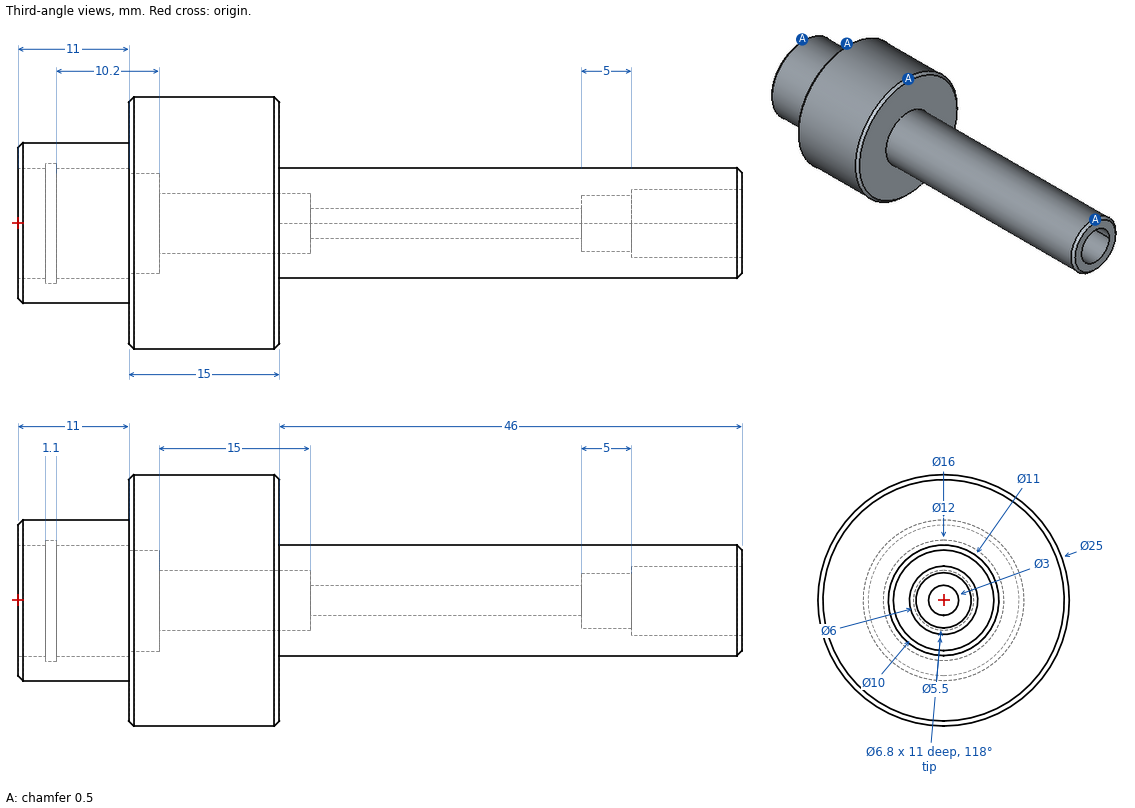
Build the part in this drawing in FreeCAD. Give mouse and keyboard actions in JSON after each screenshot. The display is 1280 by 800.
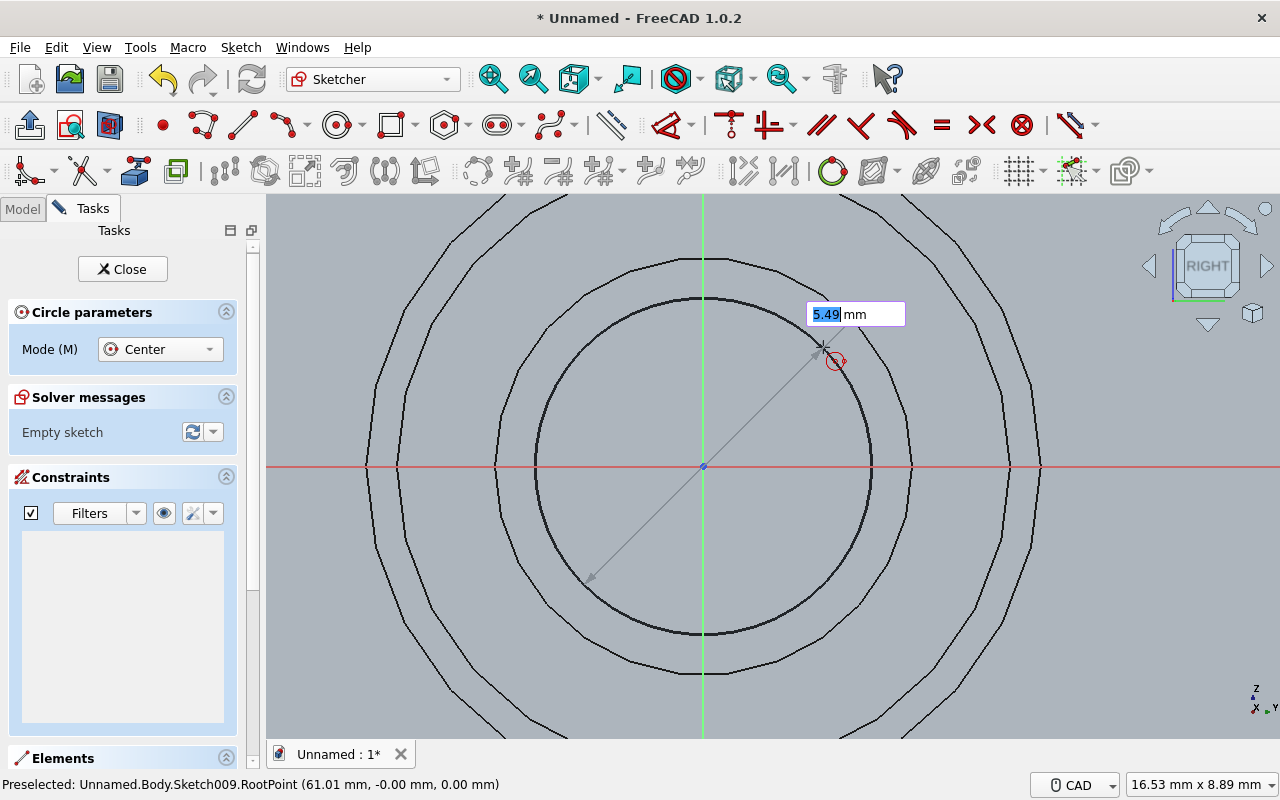
{"action": "type", "text": "5.5"}
{"action": "key", "text": "Return"}
{"action": "key", "text": "Escape"}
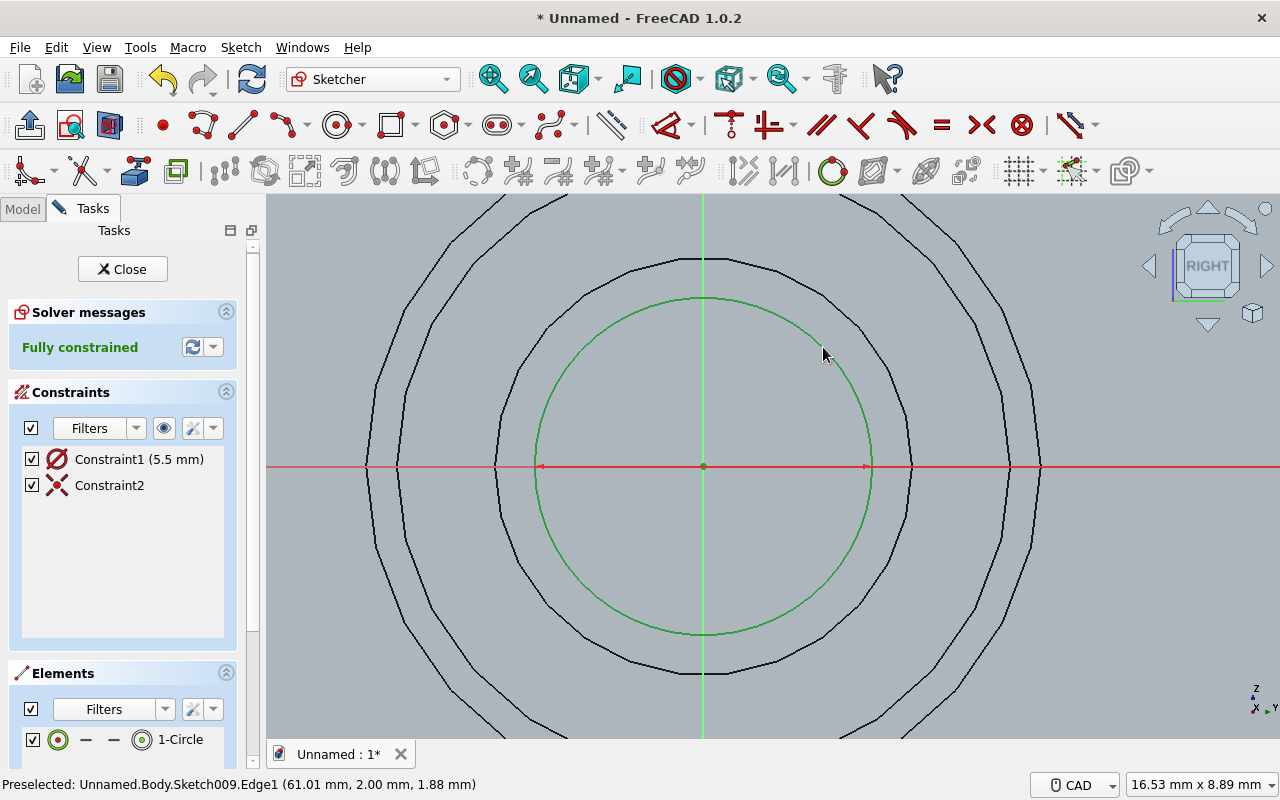
{"action": "left_click", "coordinate": [123, 269]}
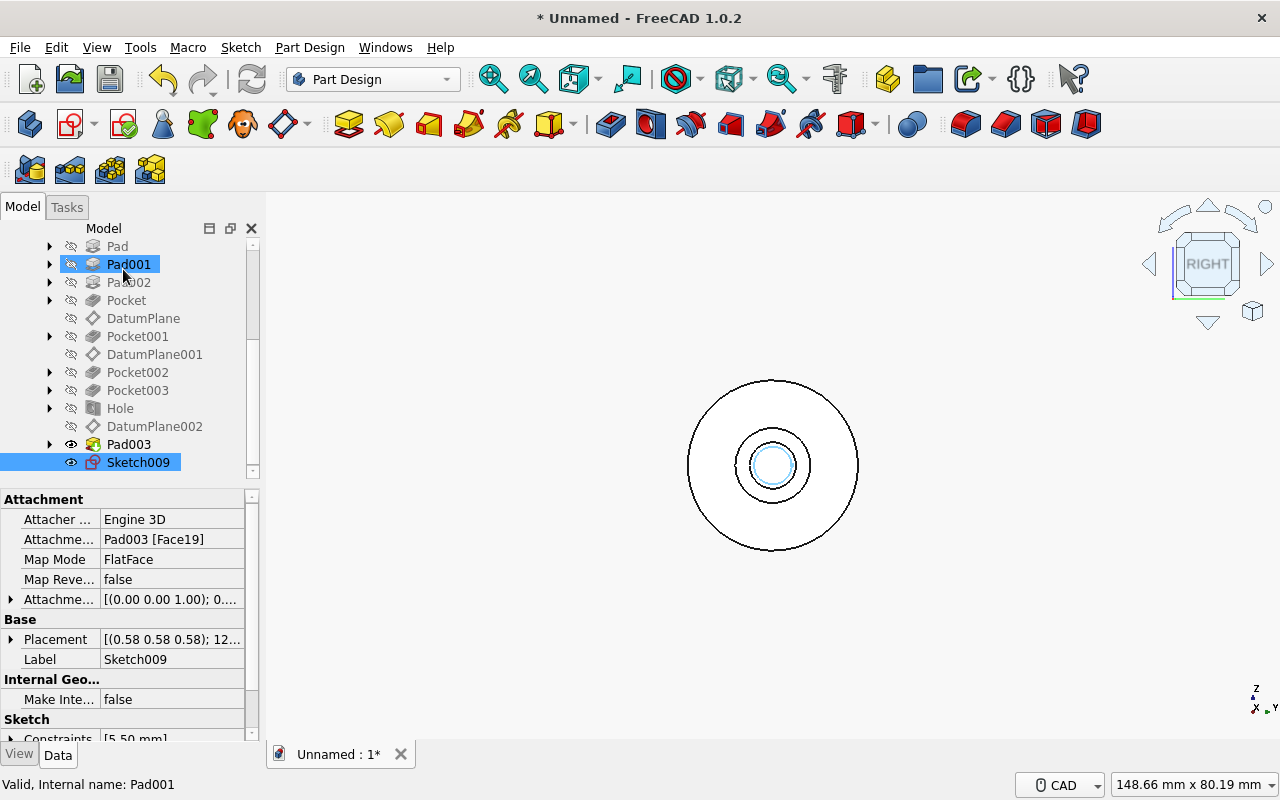
{"action": "left_click", "coordinate": [612, 124]}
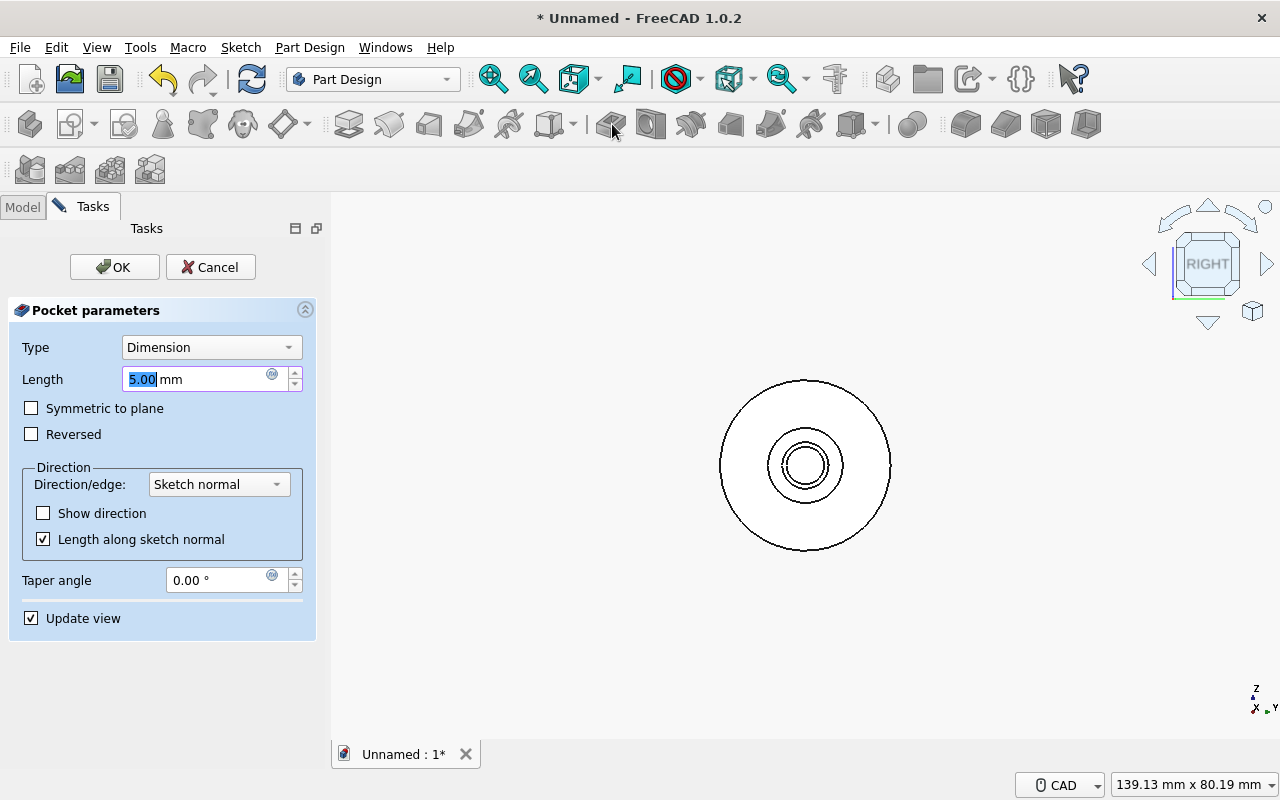
{"action": "type", "text": "5"}
{"action": "key", "text": "Tab"}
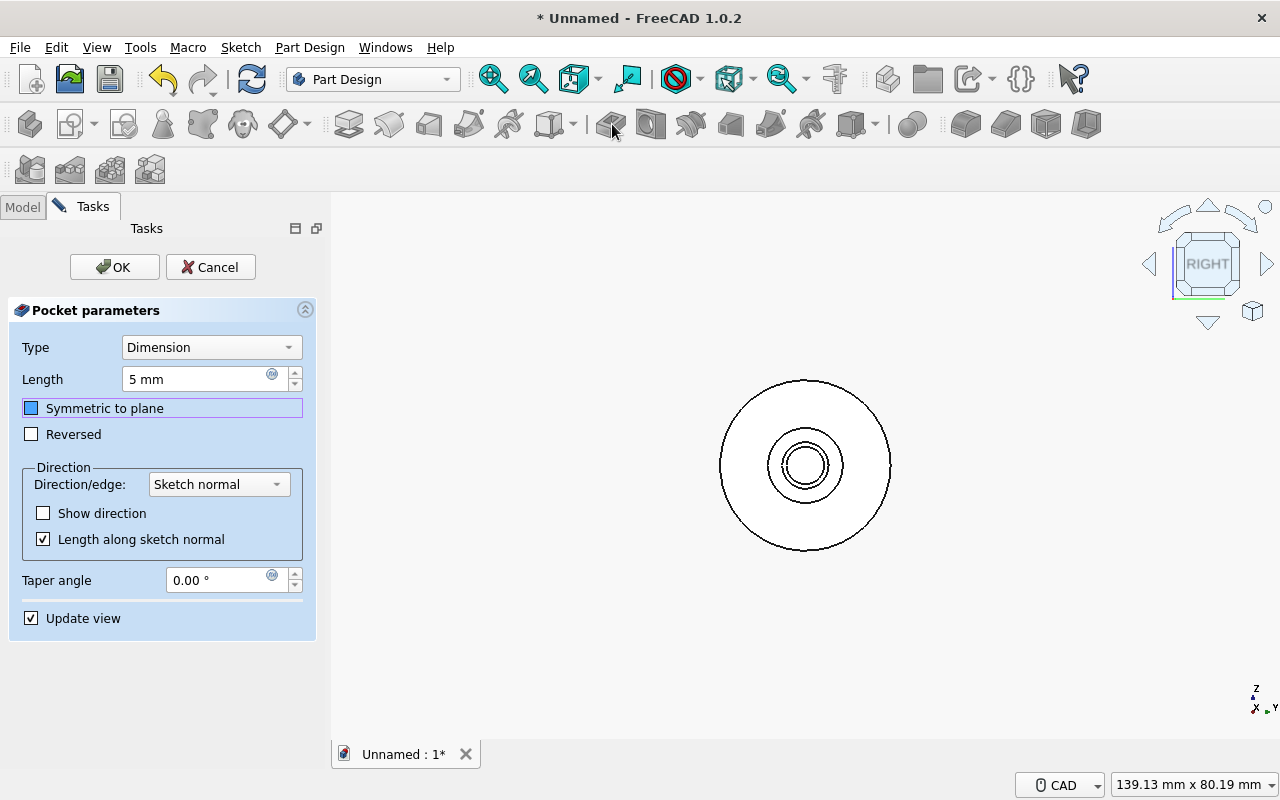
{"action": "left_click", "coordinate": [115, 267]}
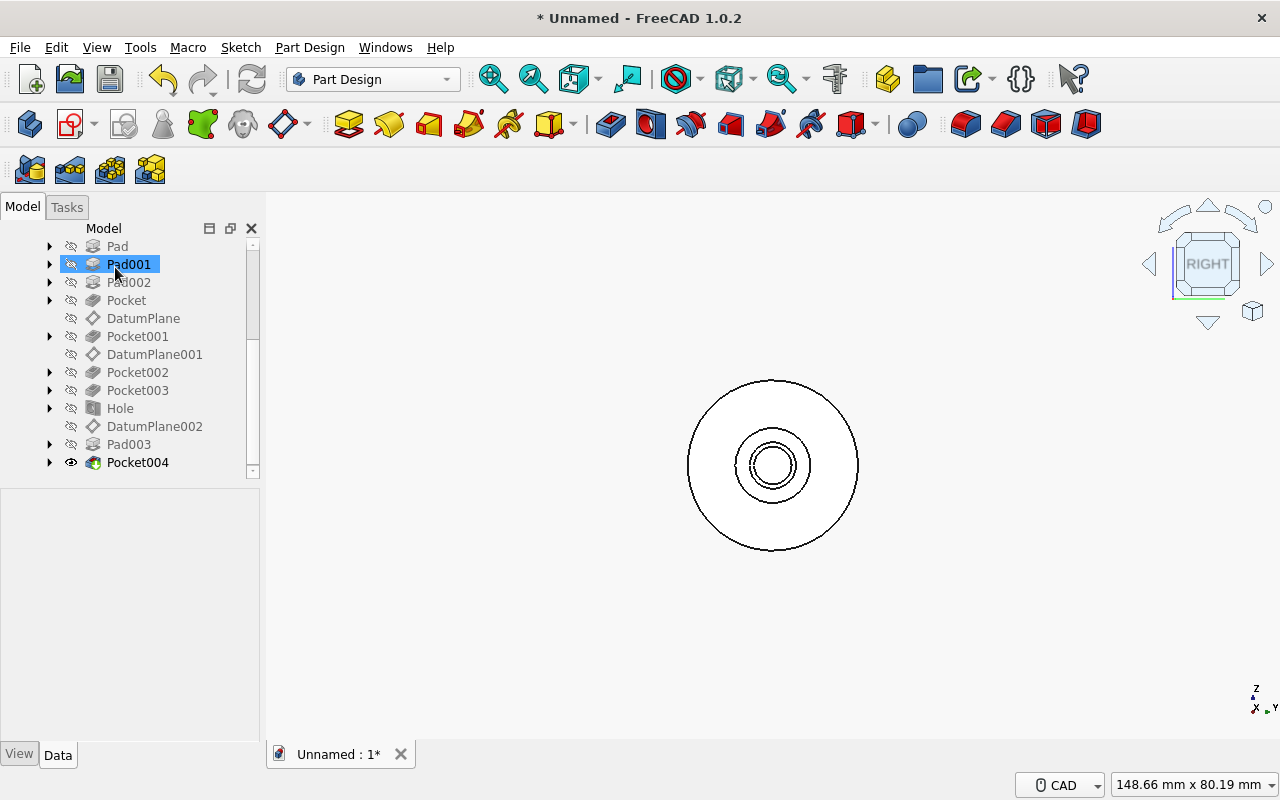
{"action": "left_click", "coordinate": [494, 80]}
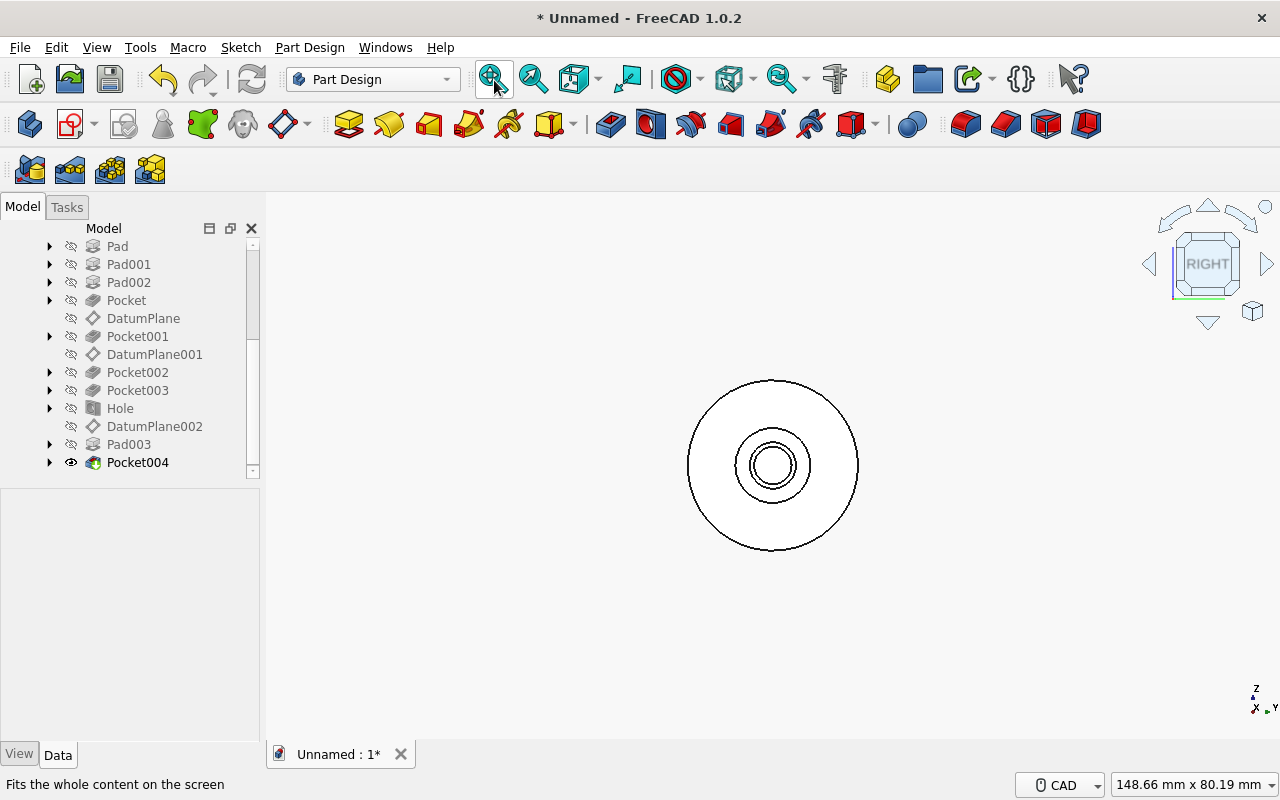
{"action": "left_click", "coordinate": [773, 464]}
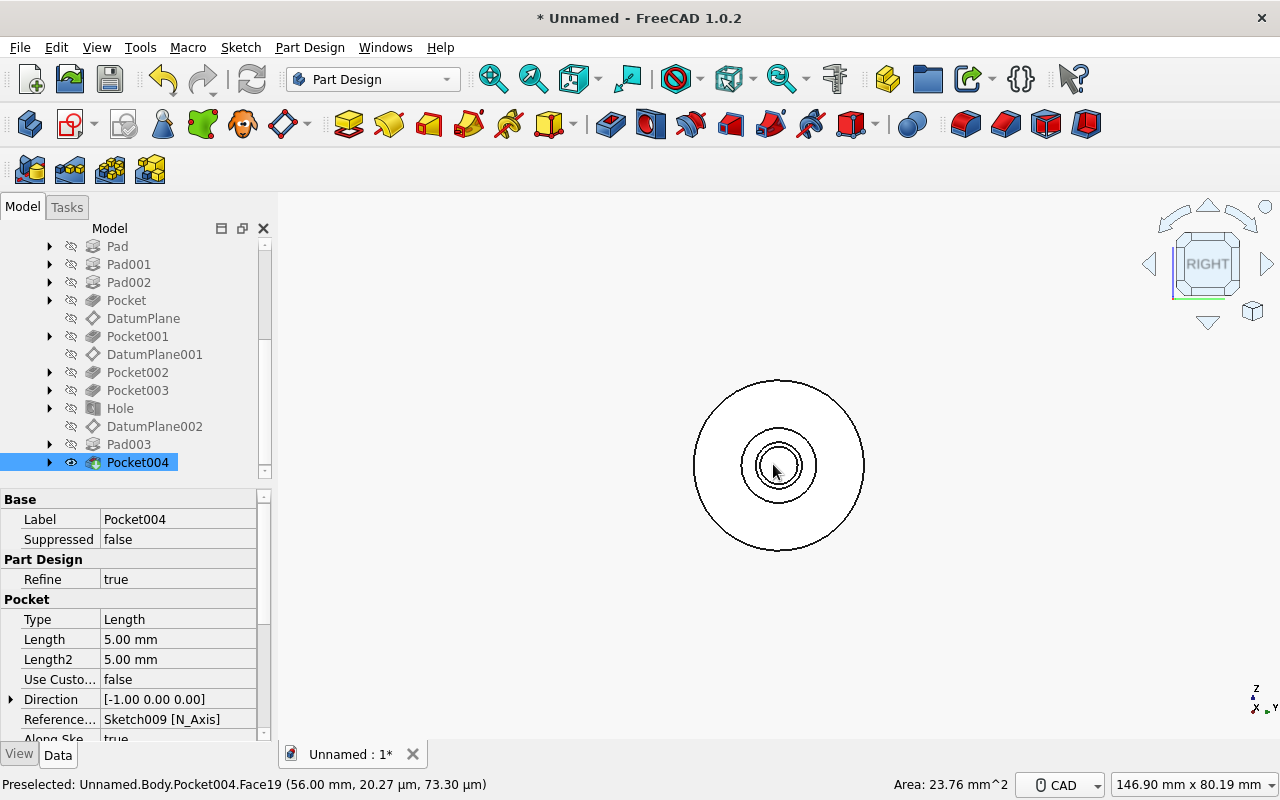
{"action": "left_click", "coordinate": [70, 124]}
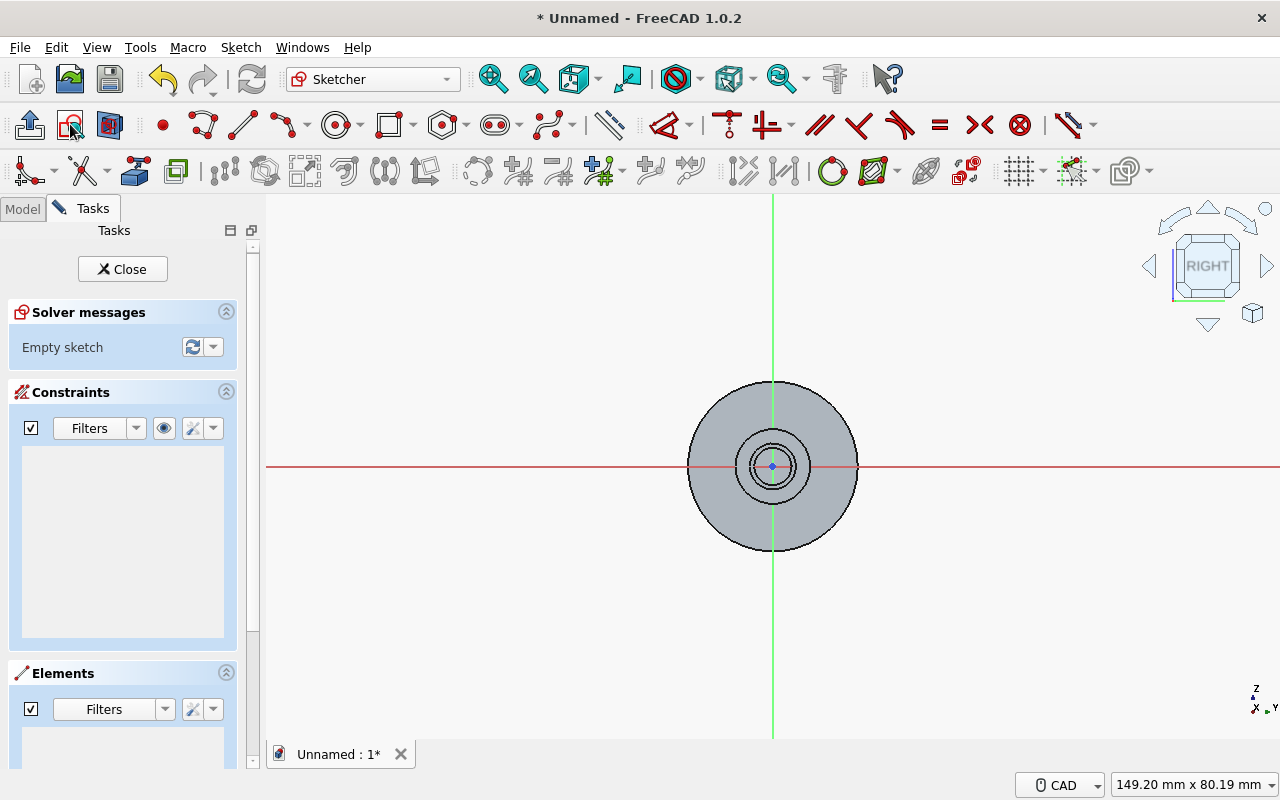
{"action": "left_click", "coordinate": [110, 126]}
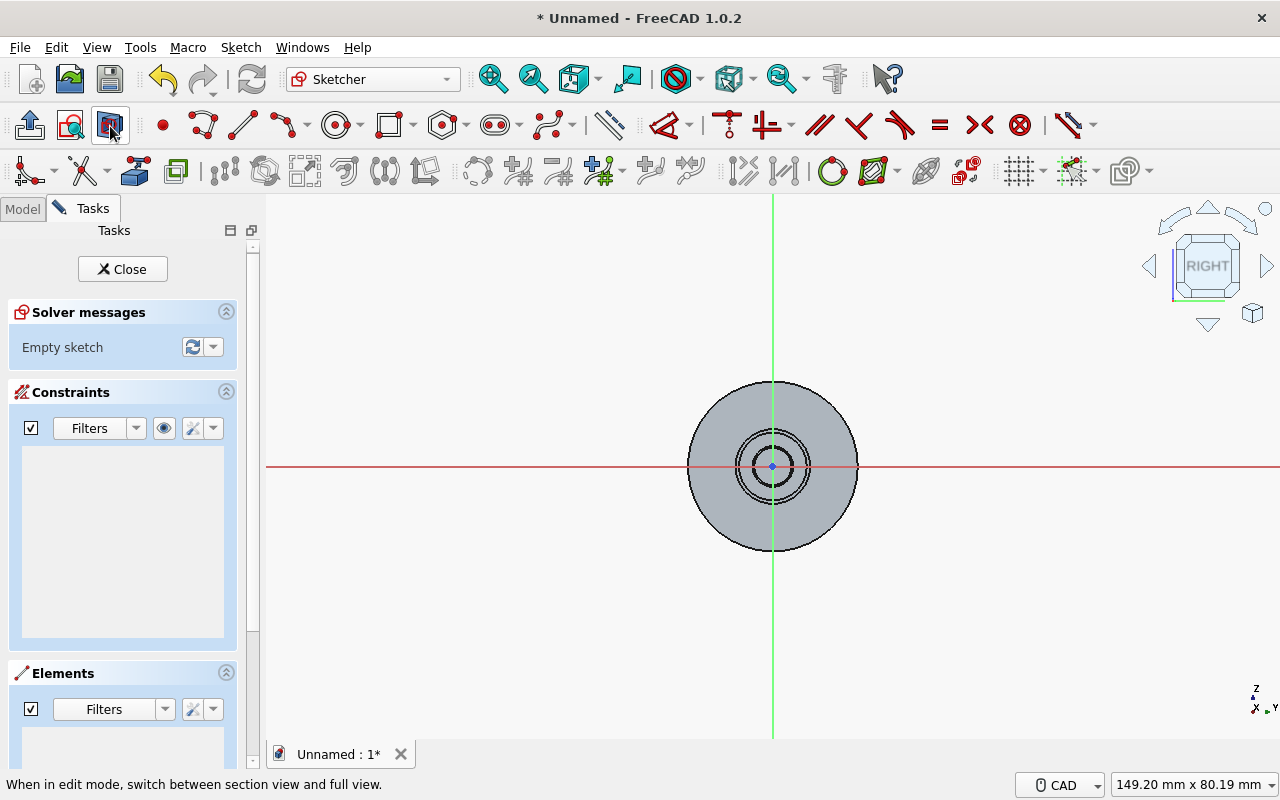
{"action": "scroll", "coordinate": [777, 466], "scroll_direction": "up", "scroll_amount": 14}